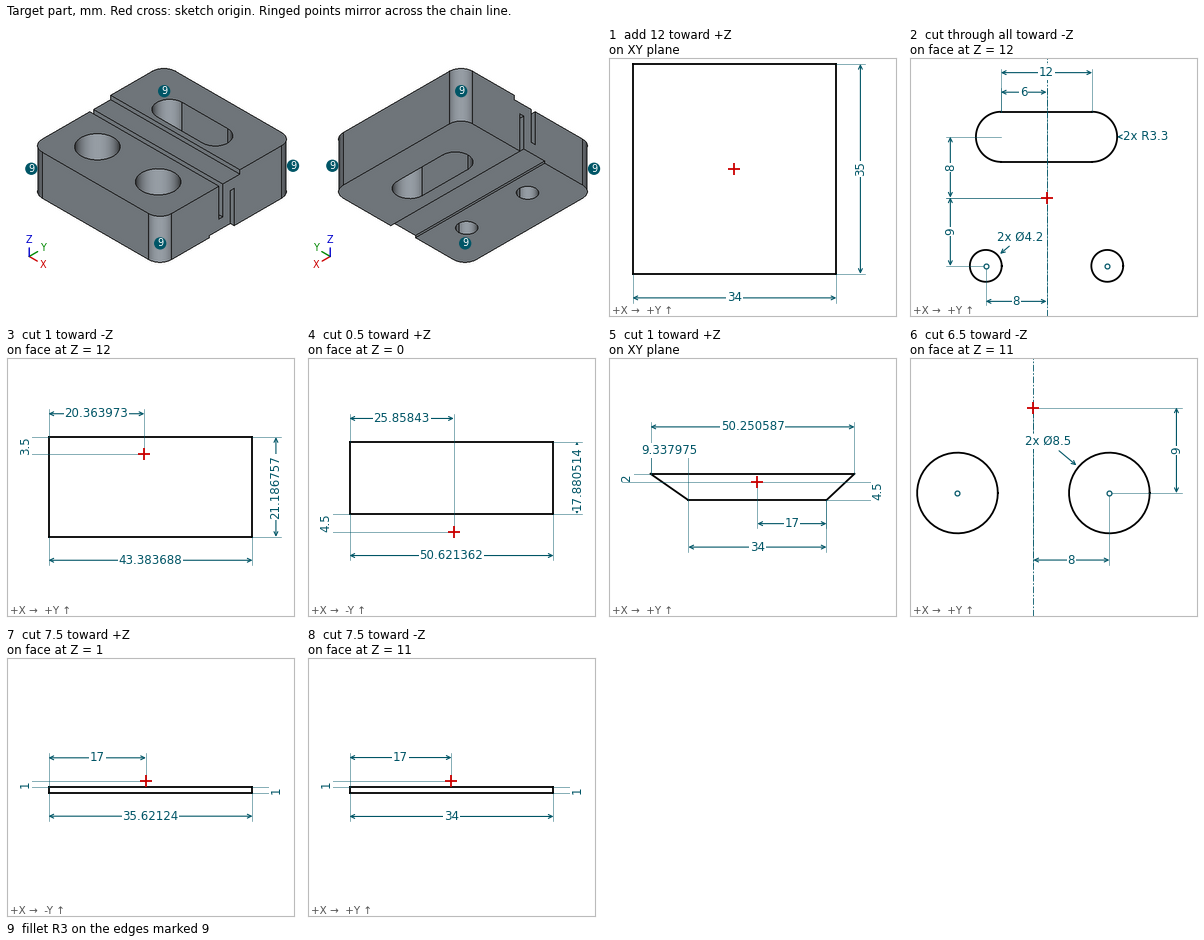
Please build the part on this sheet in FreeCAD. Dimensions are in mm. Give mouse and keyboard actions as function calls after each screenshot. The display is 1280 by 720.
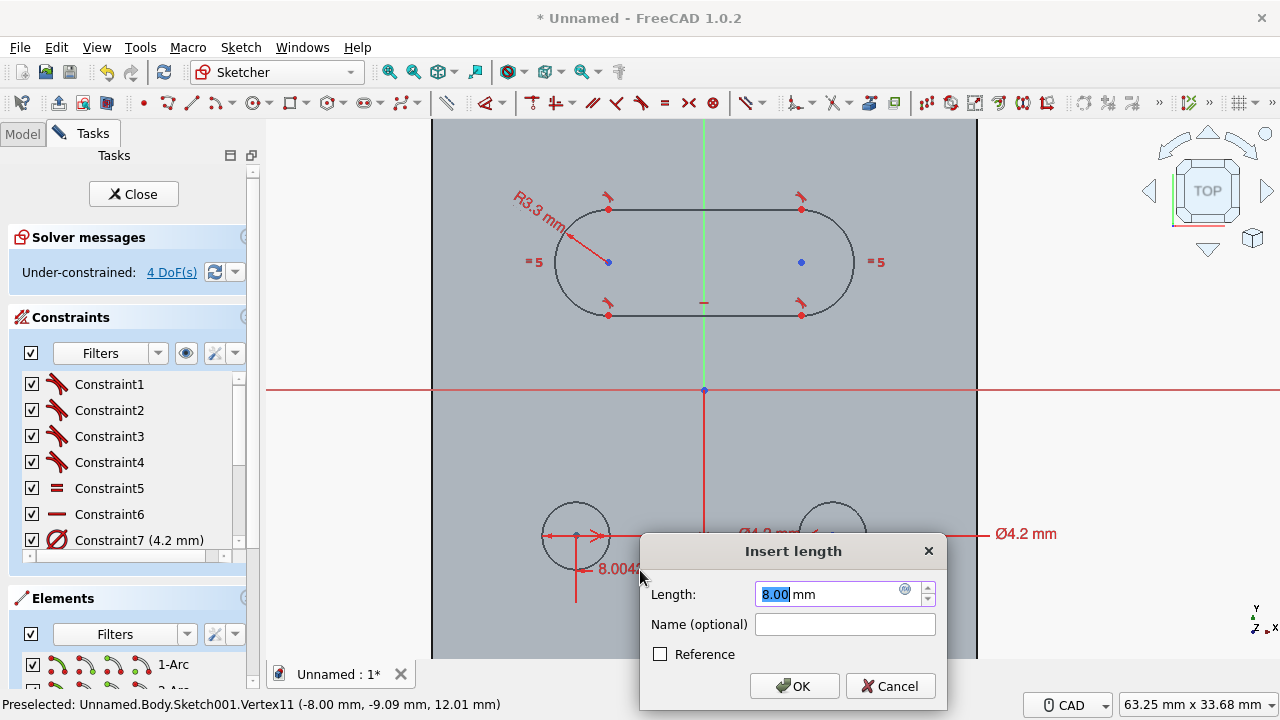
text(8)
key(Return)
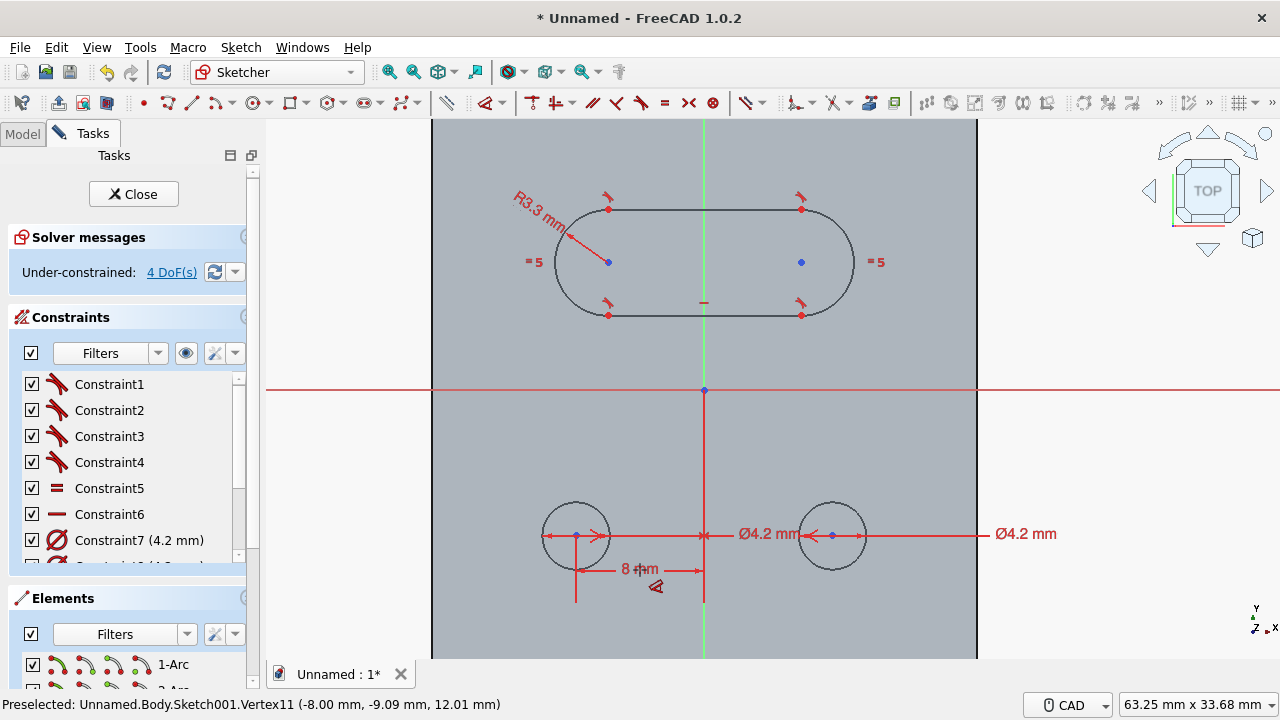
click(576, 536)
click(542, 463)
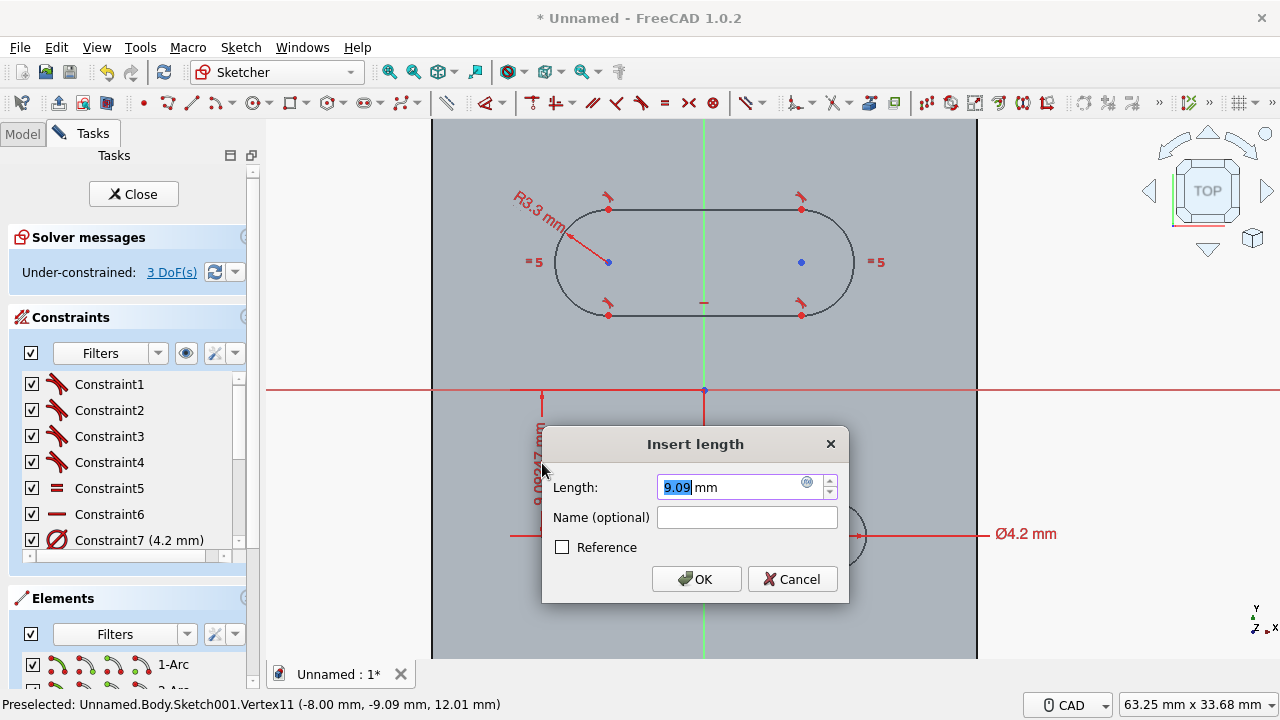
text(9)
key(Return)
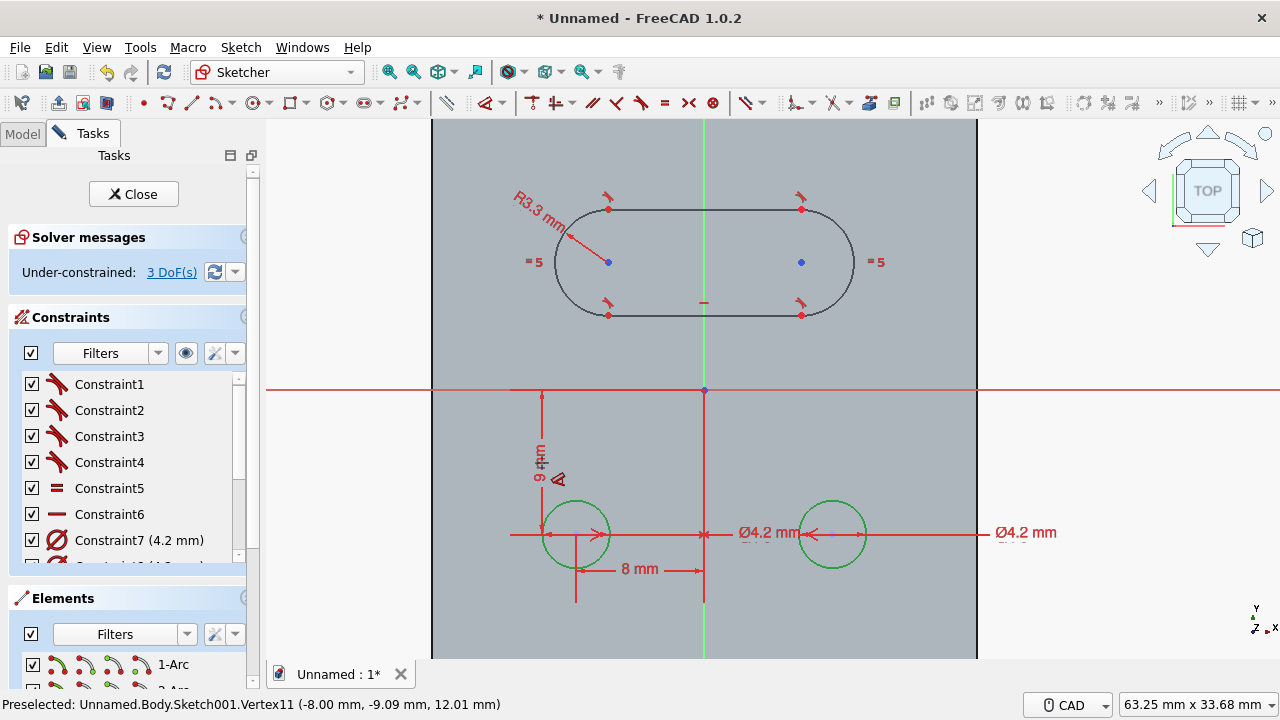
click(666, 210)
click(660, 176)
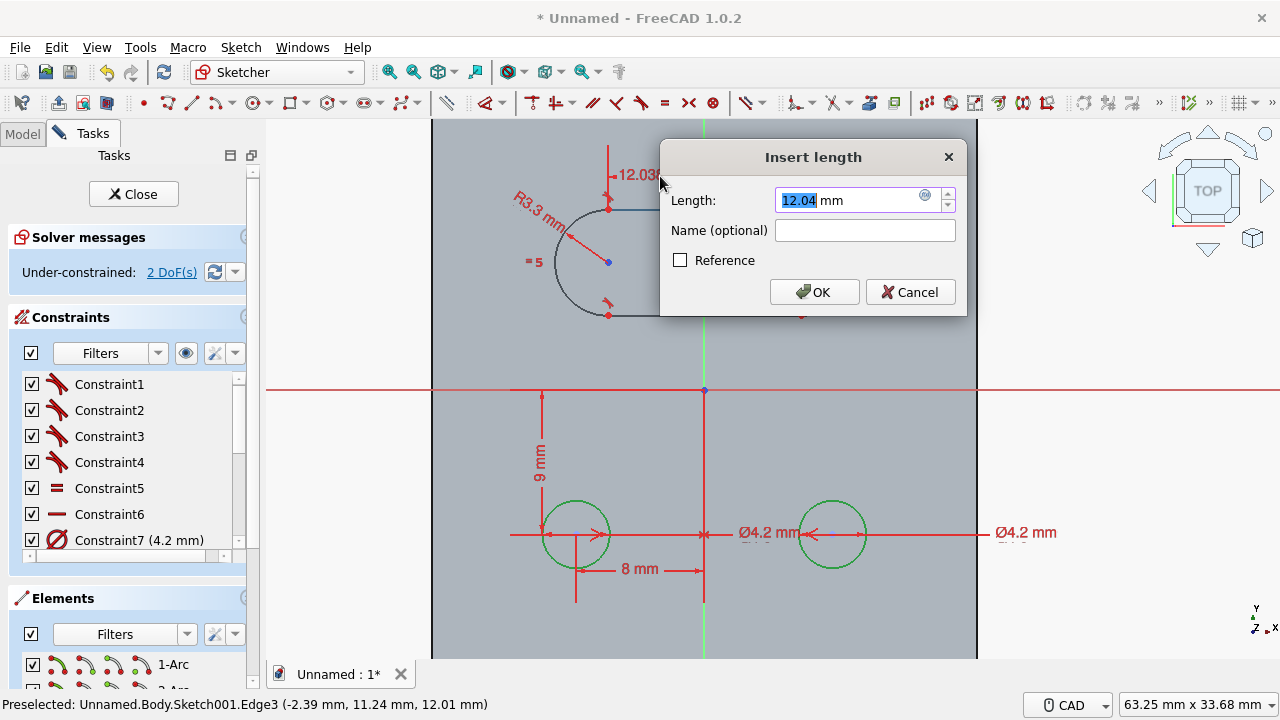
text(12)
key(Return)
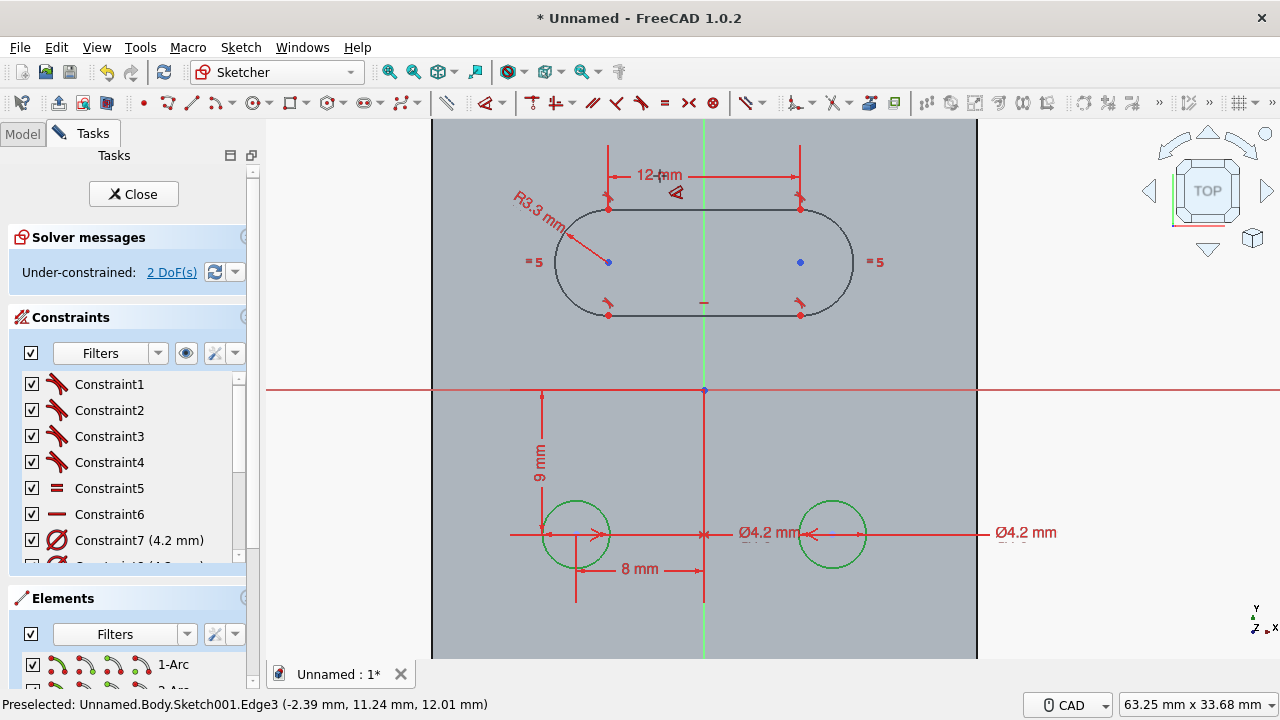
click(608, 210)
click(656, 424)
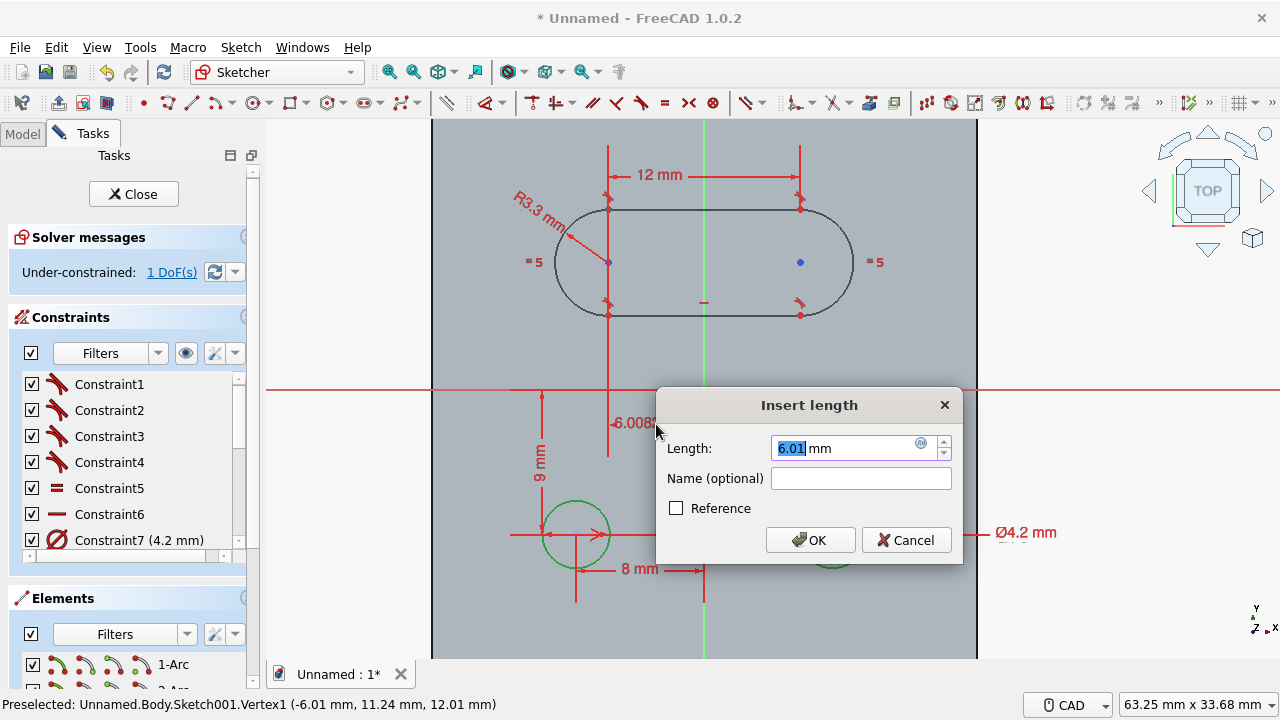
text(6)
key(Return)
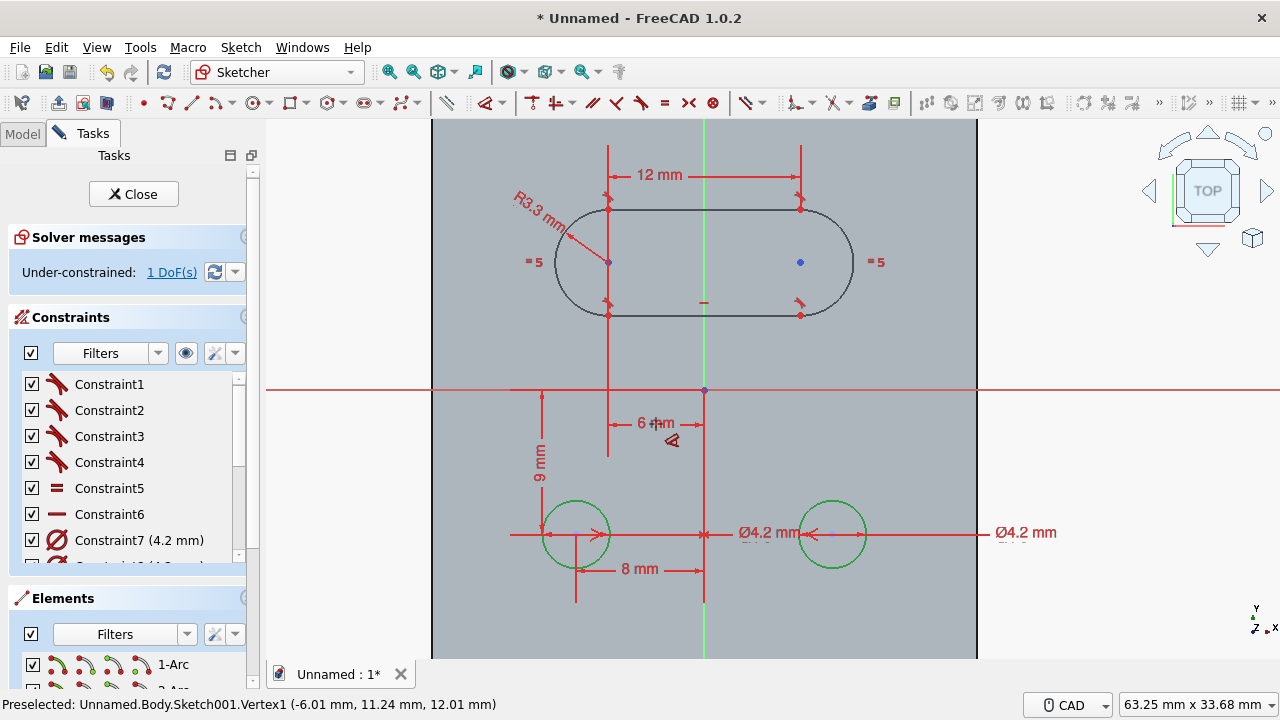
click(608, 263)
click(574, 327)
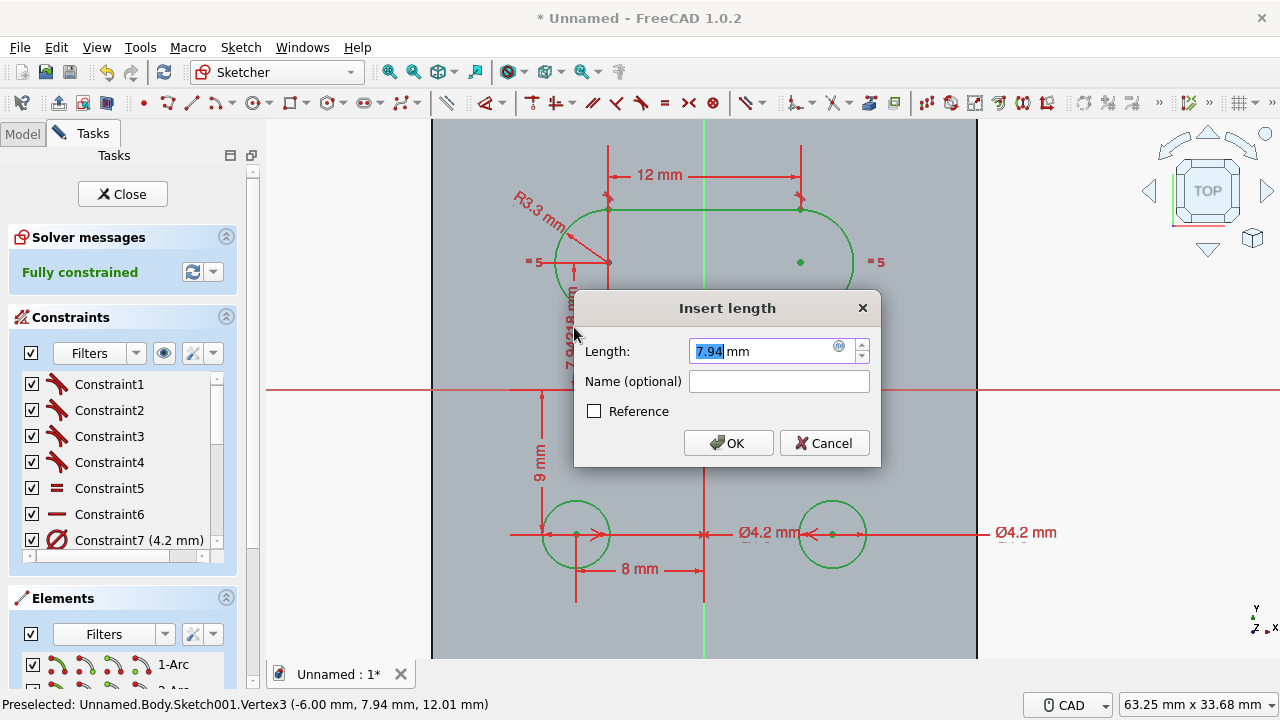
text(8)
key(Return)
key(Escape)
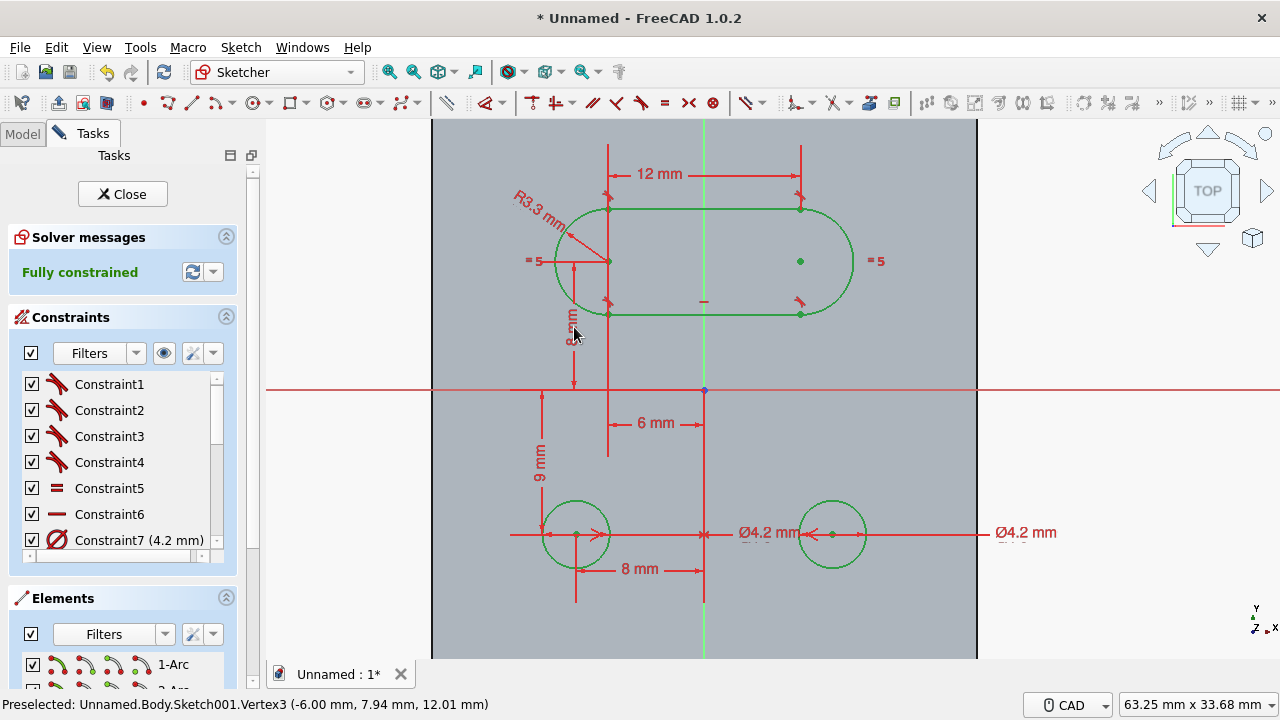
click(123, 194)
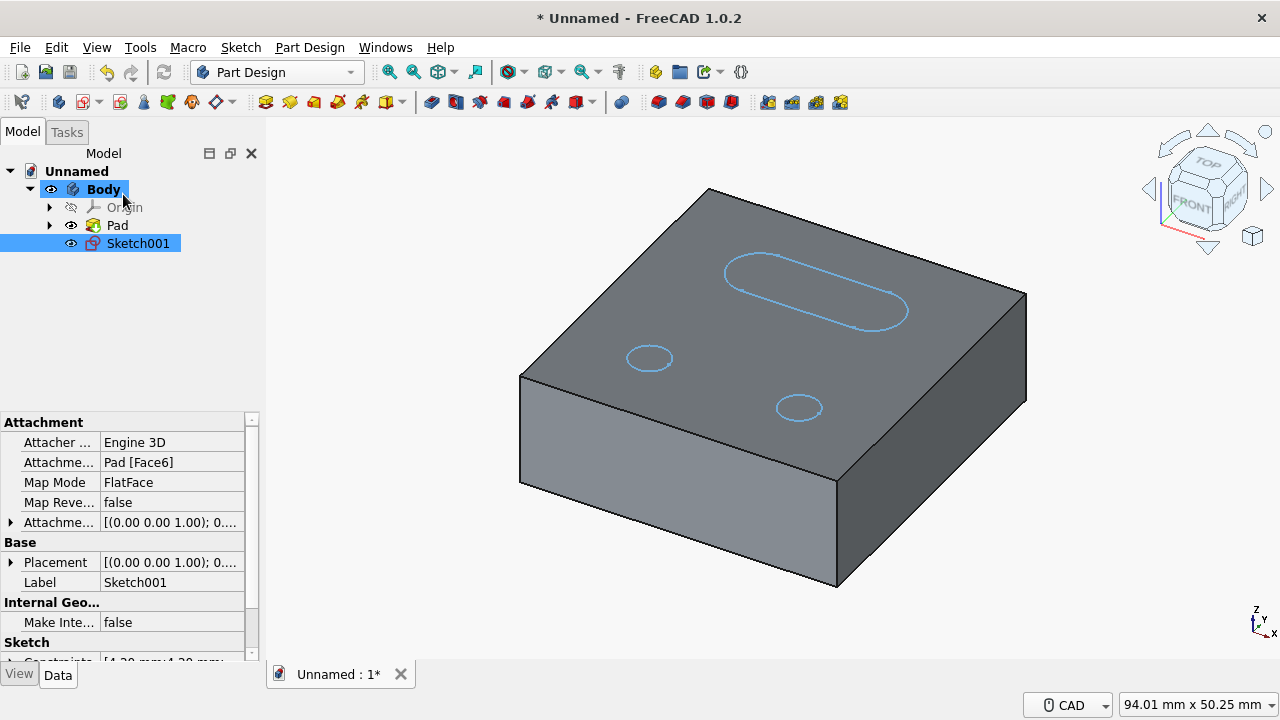
click(432, 102)